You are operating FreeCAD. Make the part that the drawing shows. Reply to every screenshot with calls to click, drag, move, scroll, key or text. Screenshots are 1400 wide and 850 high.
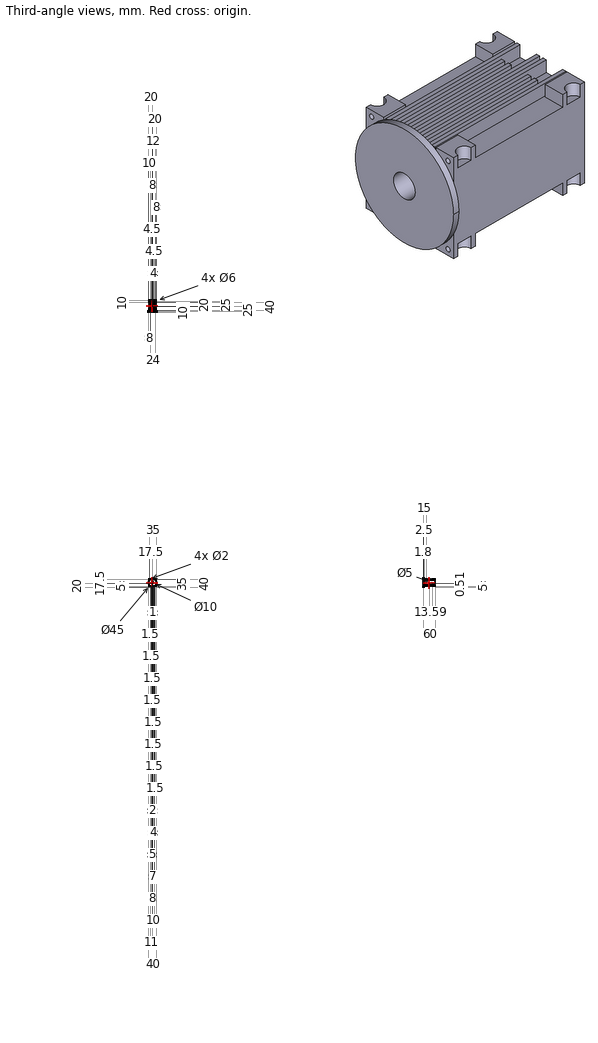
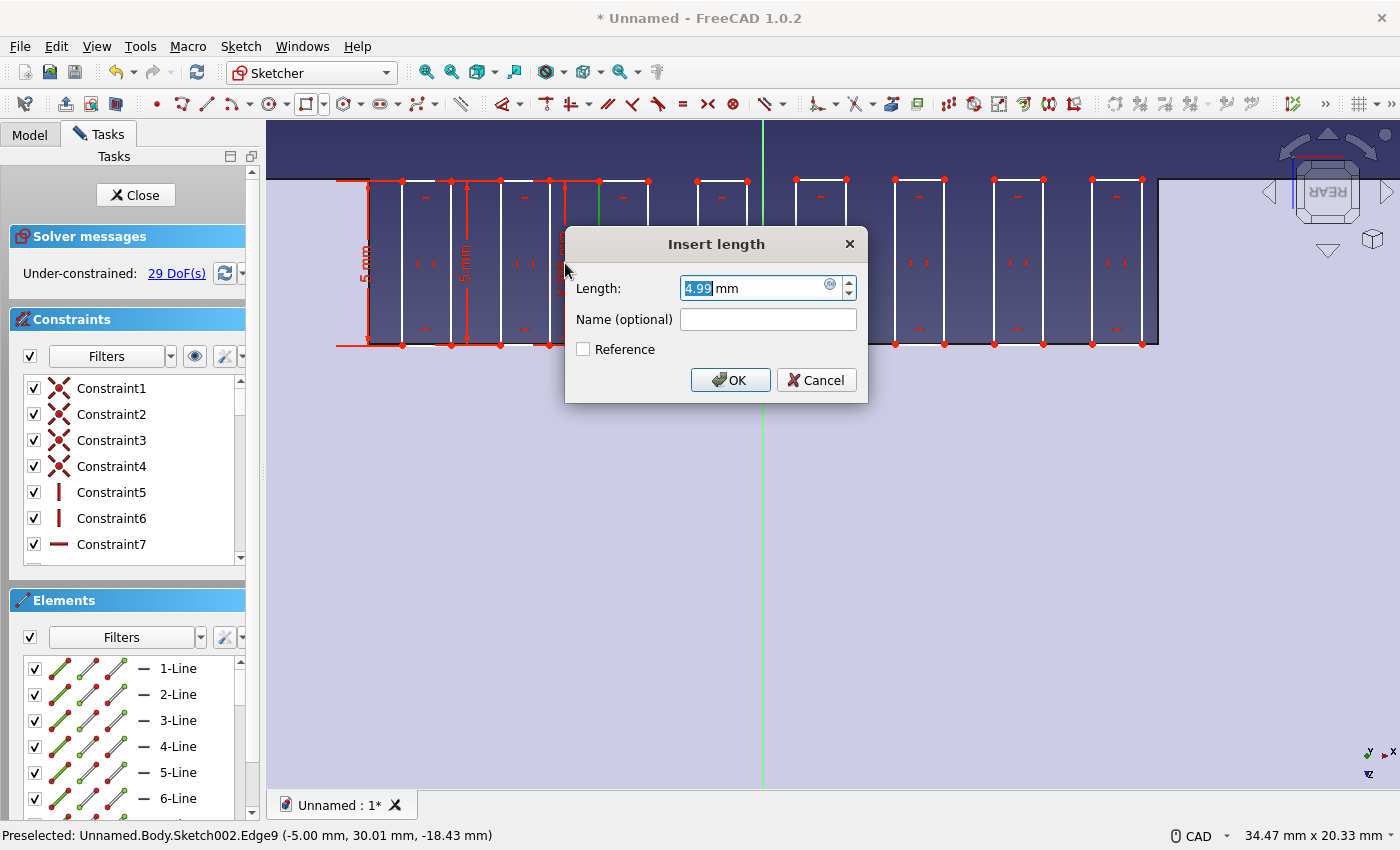
text(5)
key(Return)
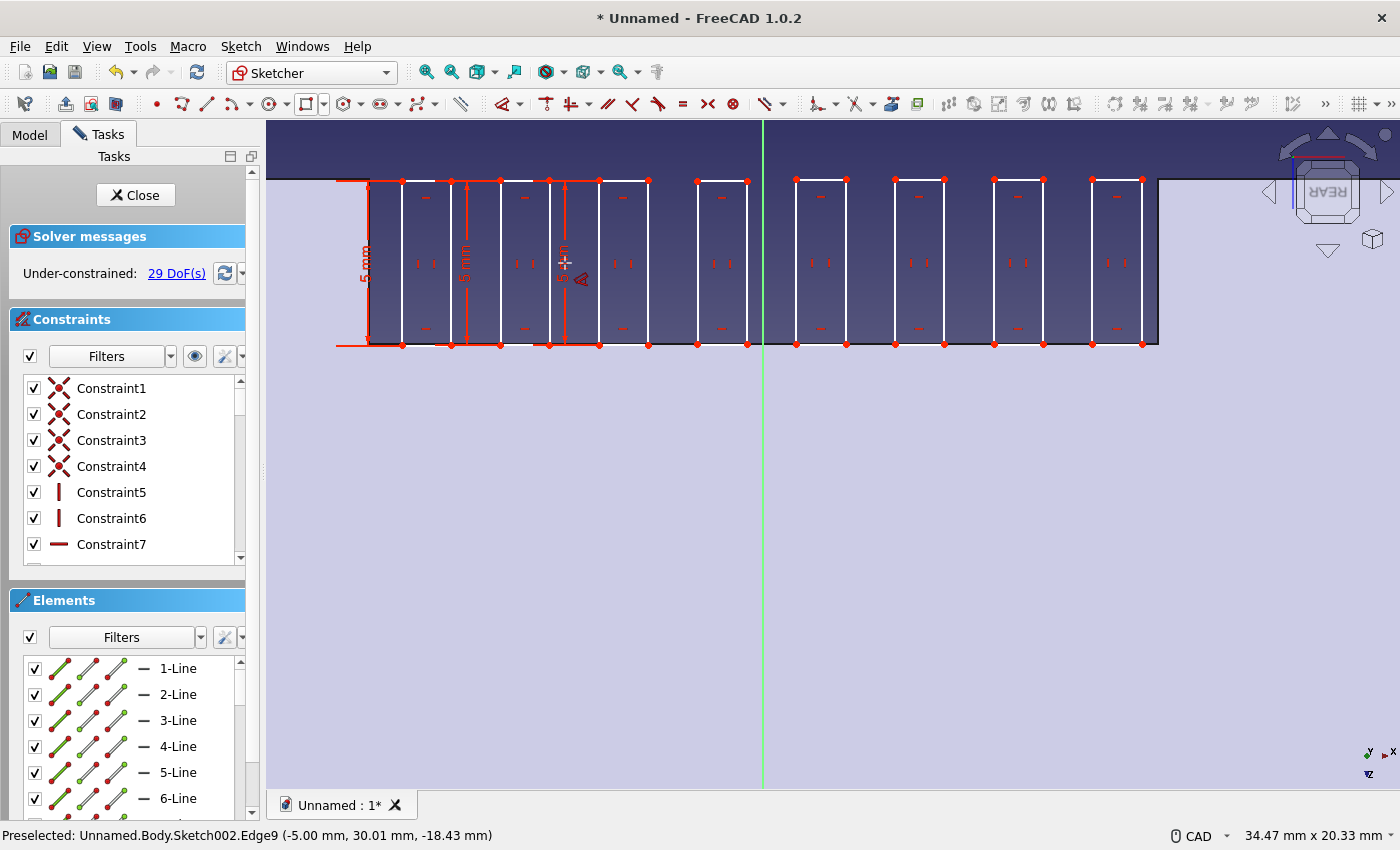
click(698, 230)
click(664, 263)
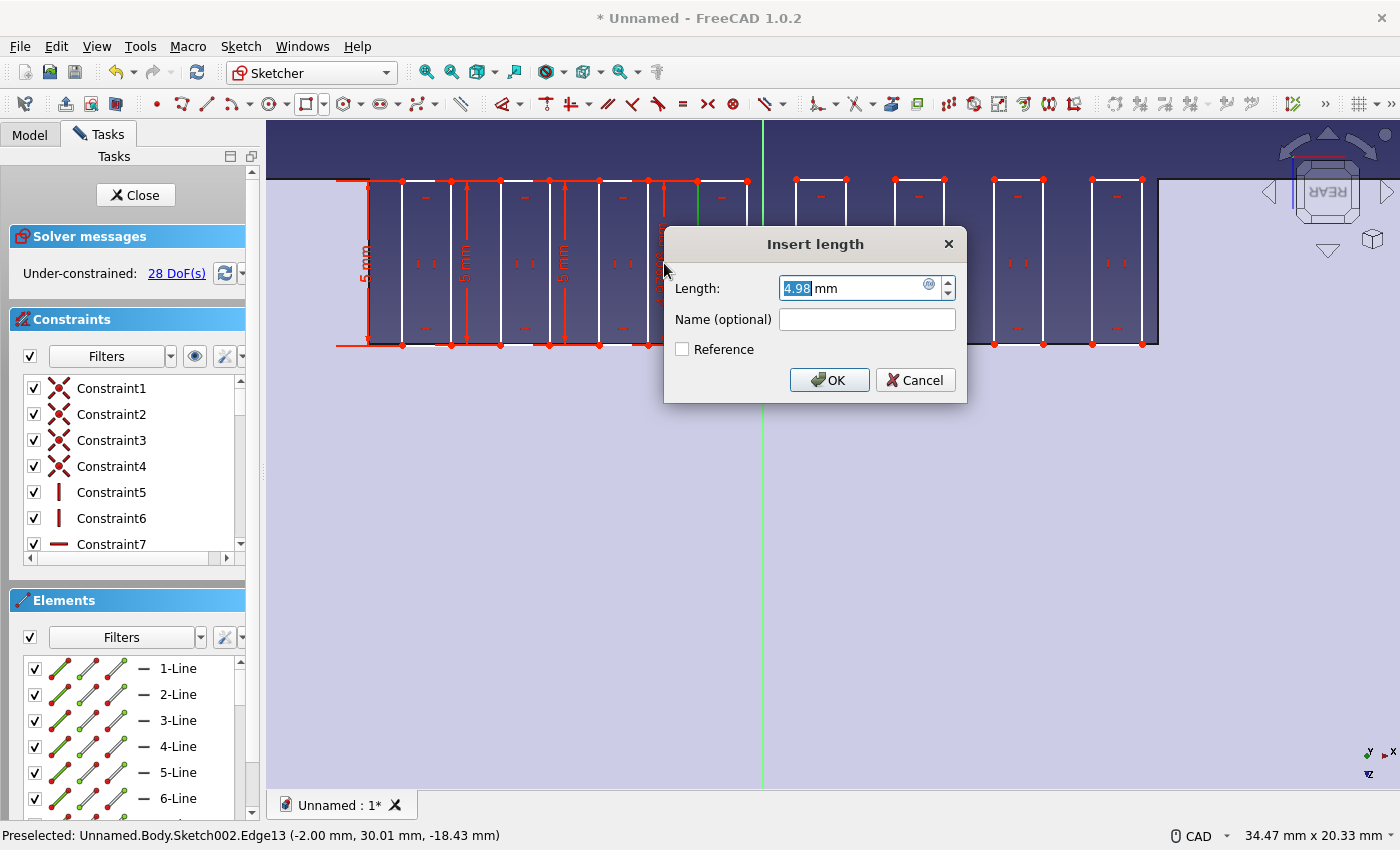
text(5)
key(Return)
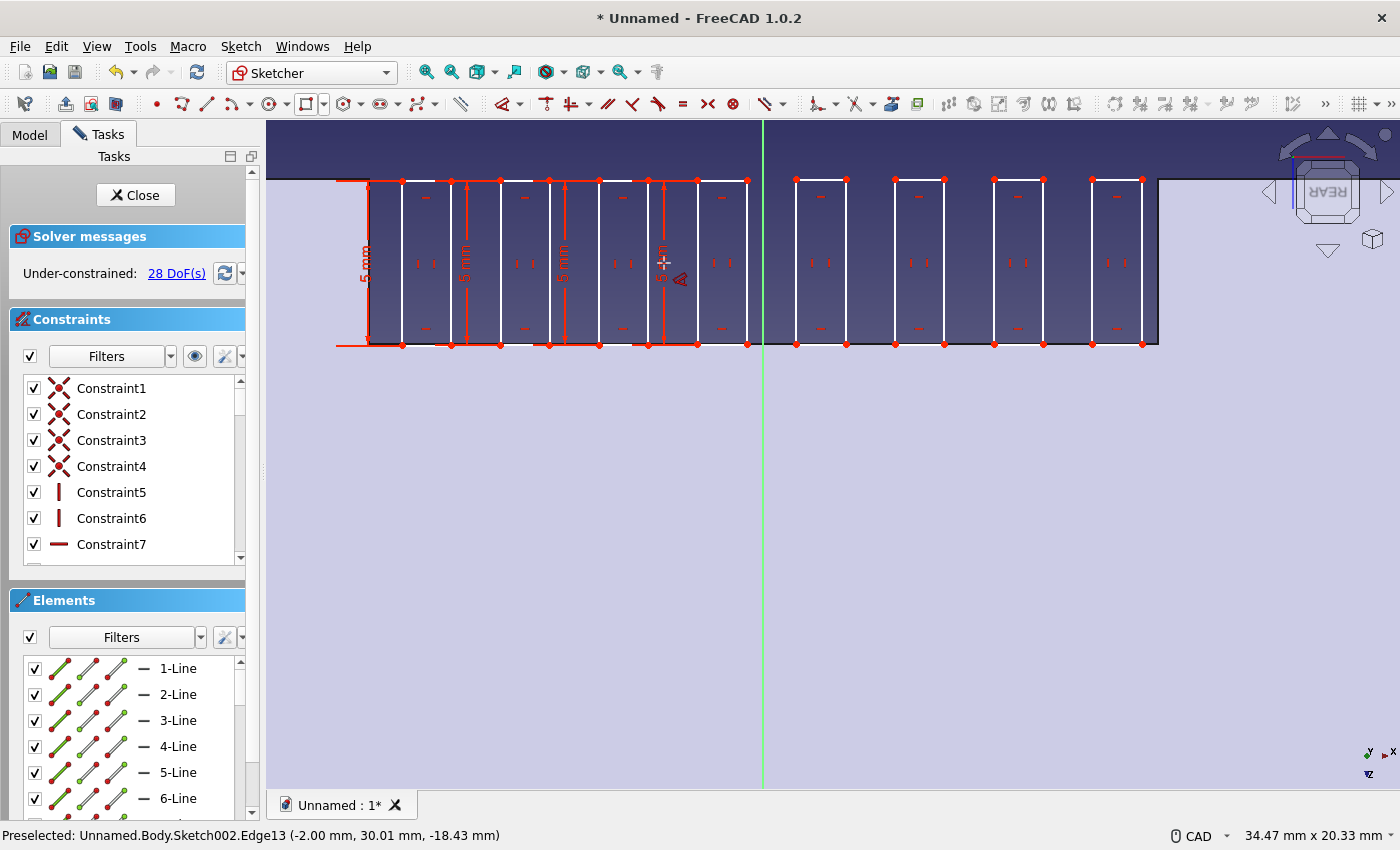
click(796, 229)
click(830, 262)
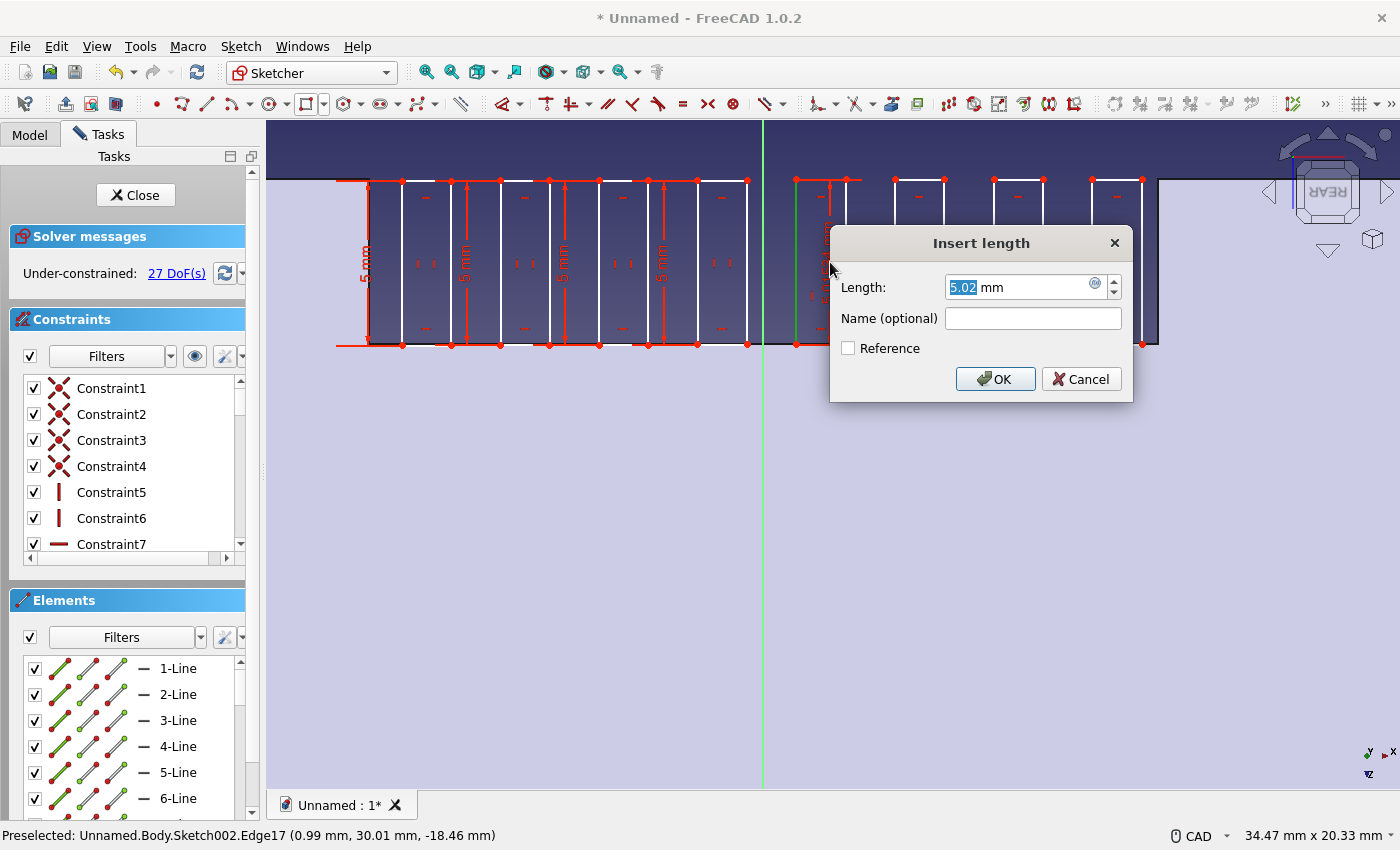
text(5)
key(Return)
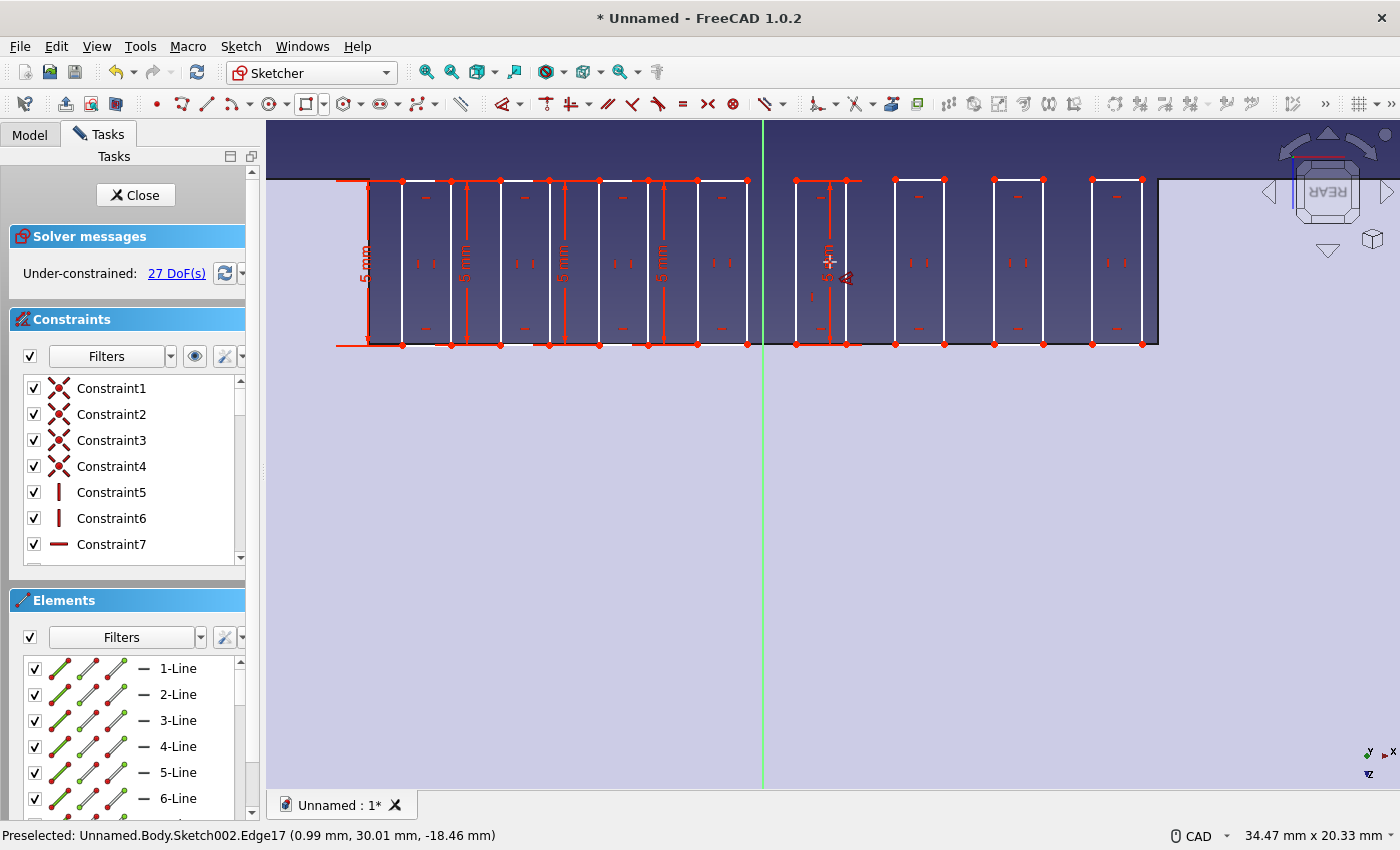
click(895, 229)
click(929, 262)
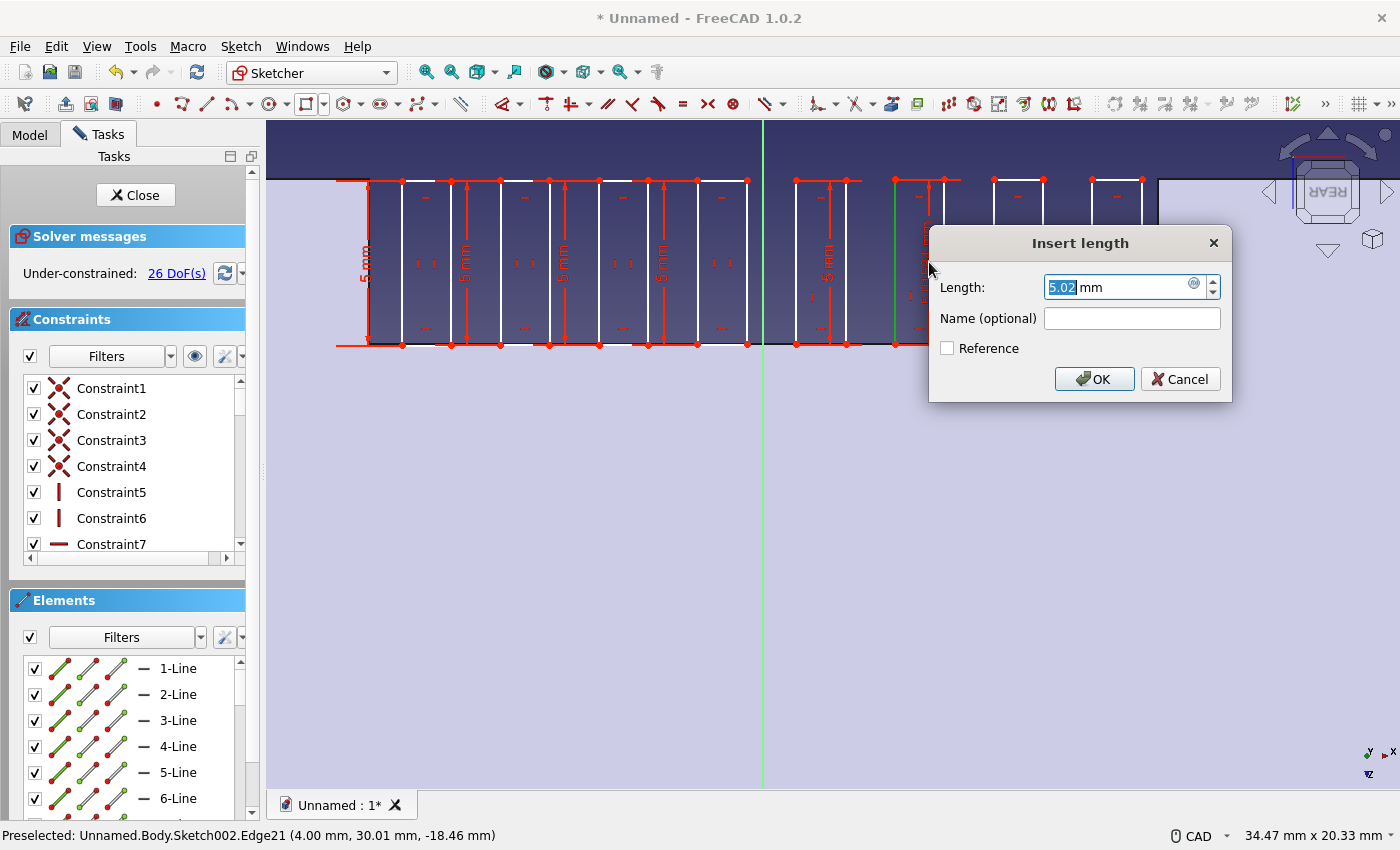
text(5)
key(Return)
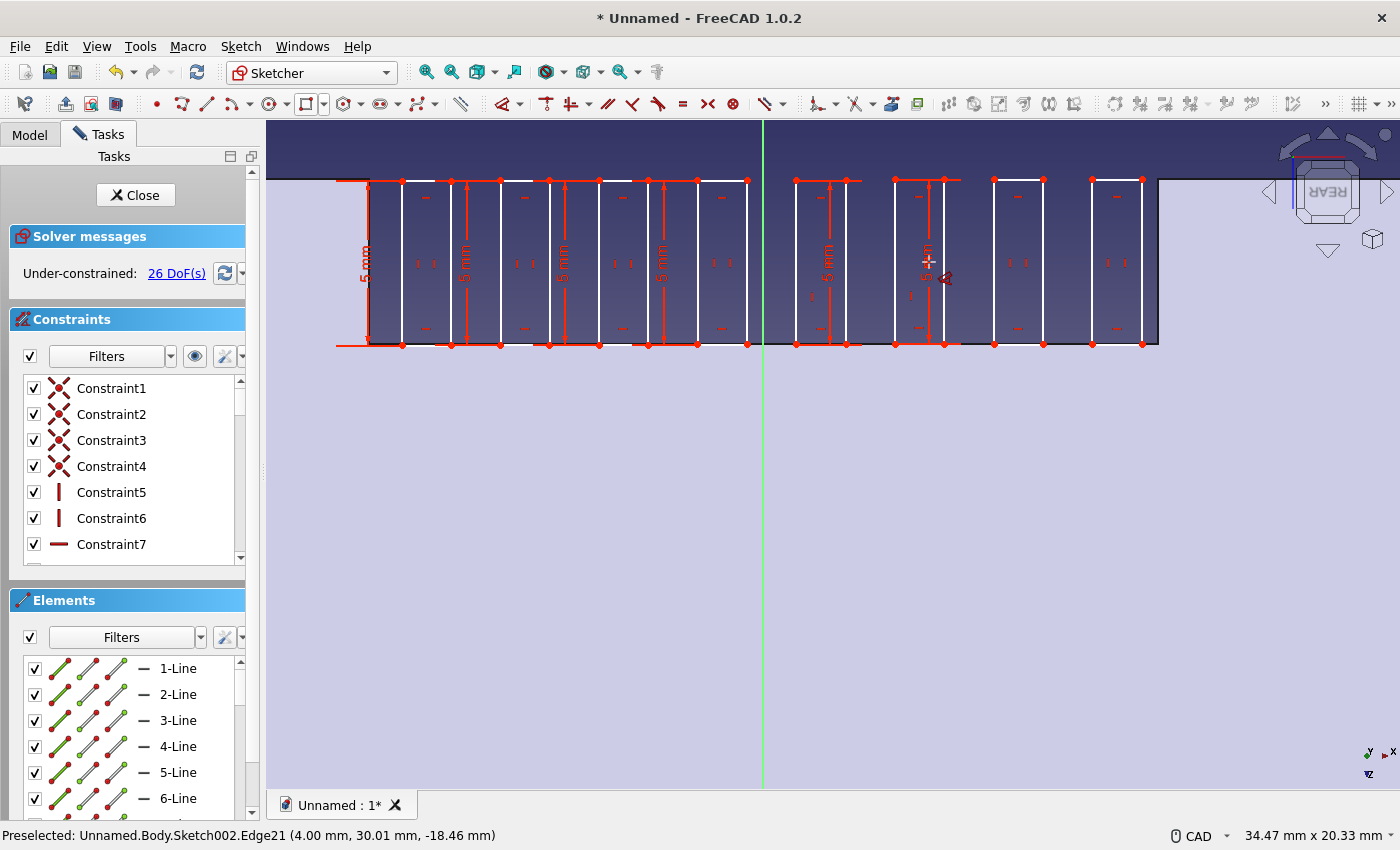
click(994, 229)
click(1028, 262)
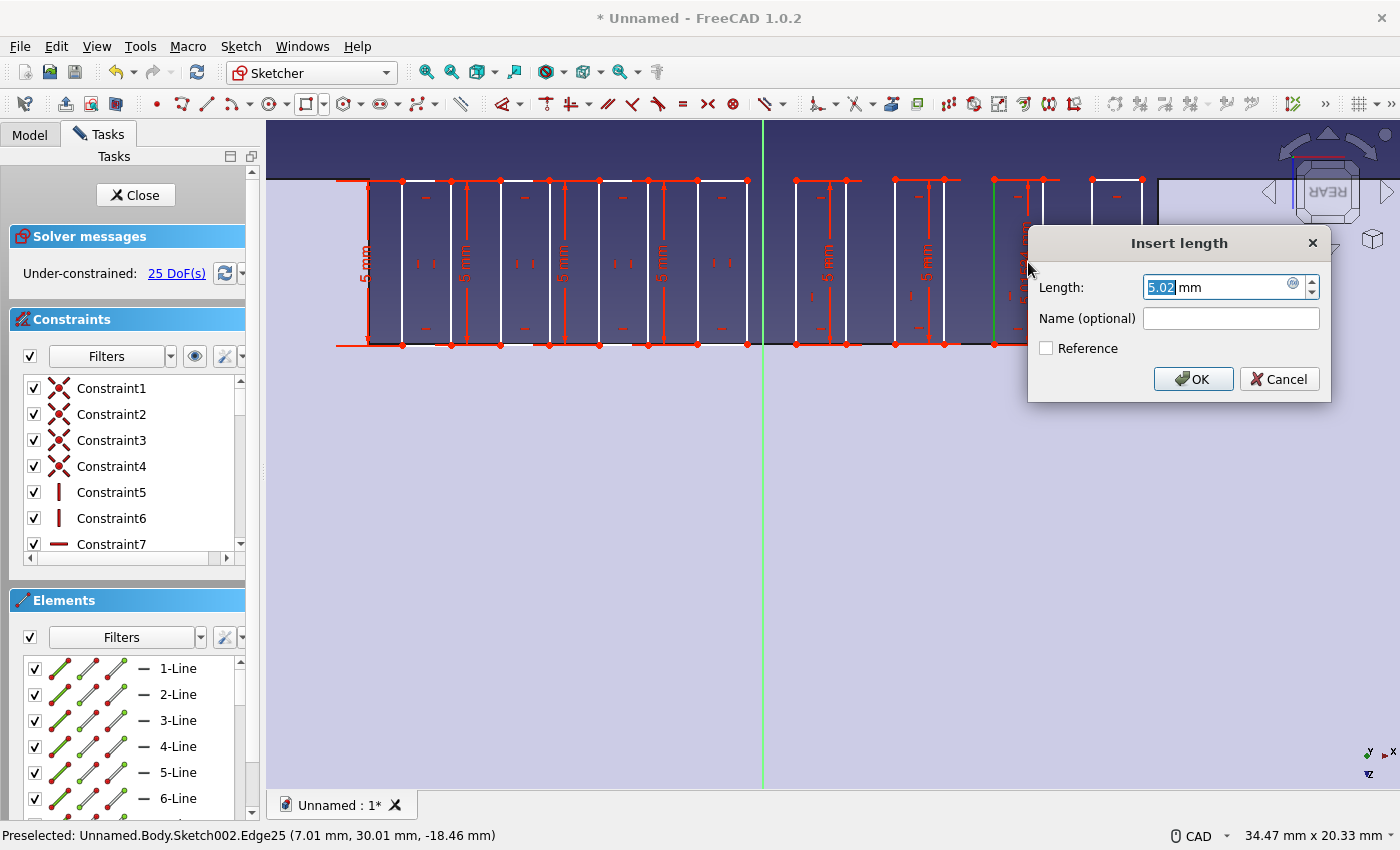
text(5)
key(Return)